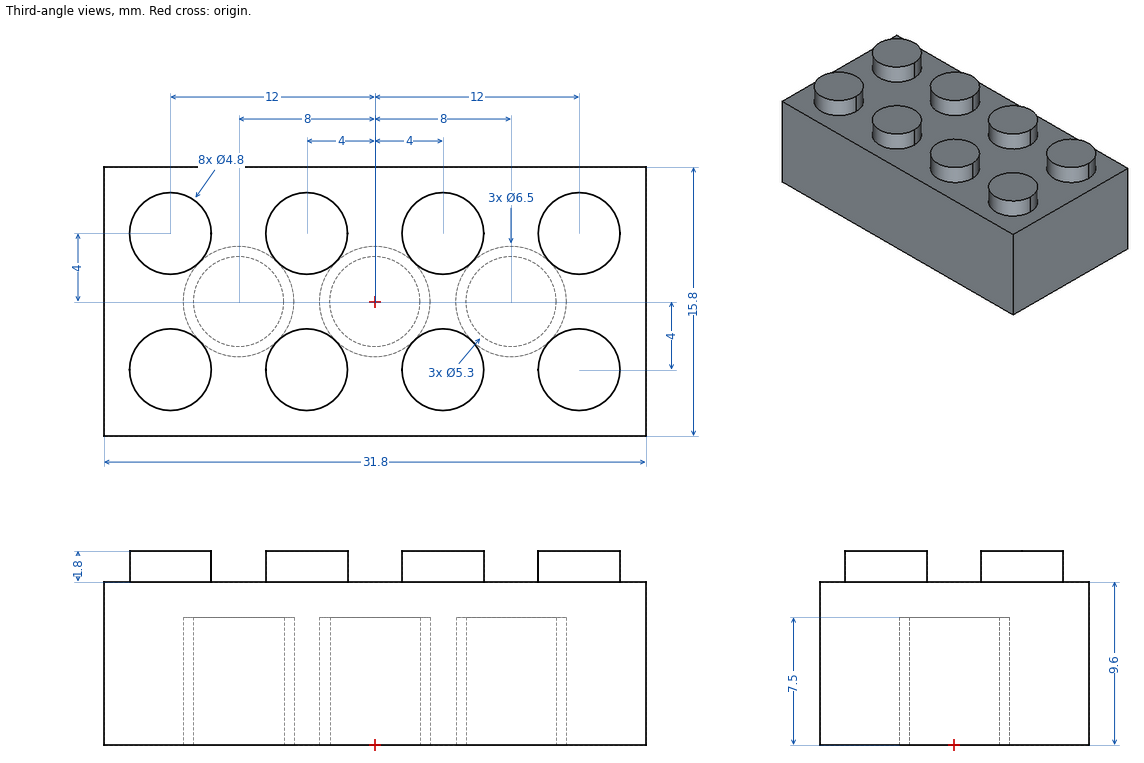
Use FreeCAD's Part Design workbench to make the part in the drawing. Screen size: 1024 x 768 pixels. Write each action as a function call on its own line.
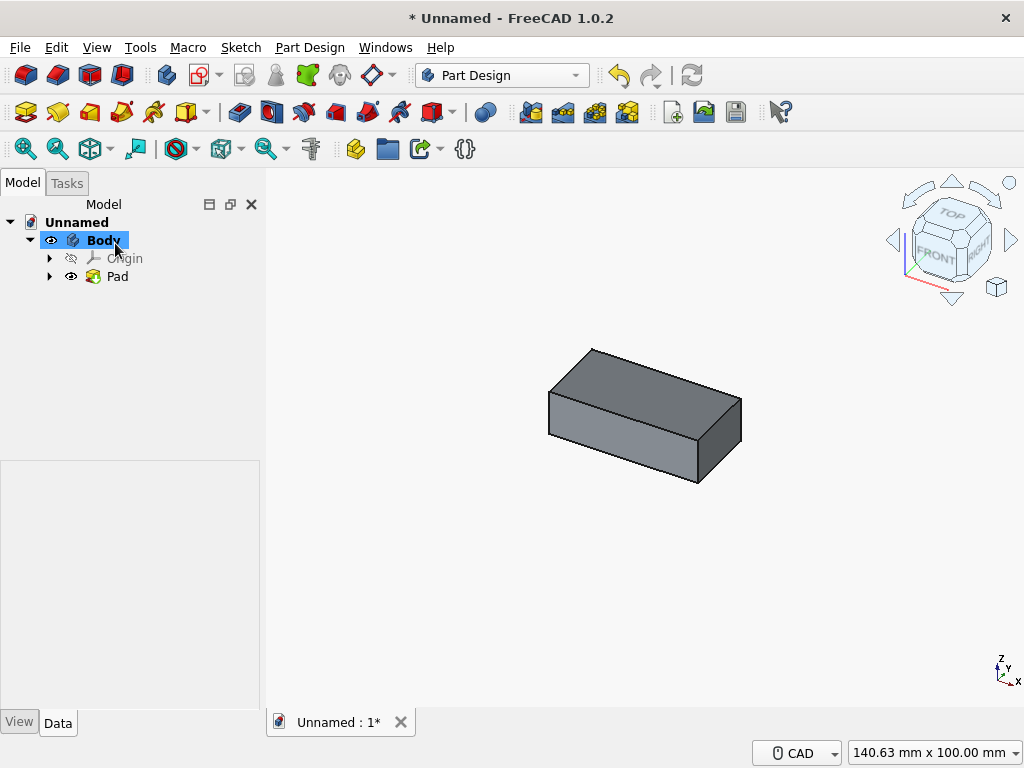
click(26, 150)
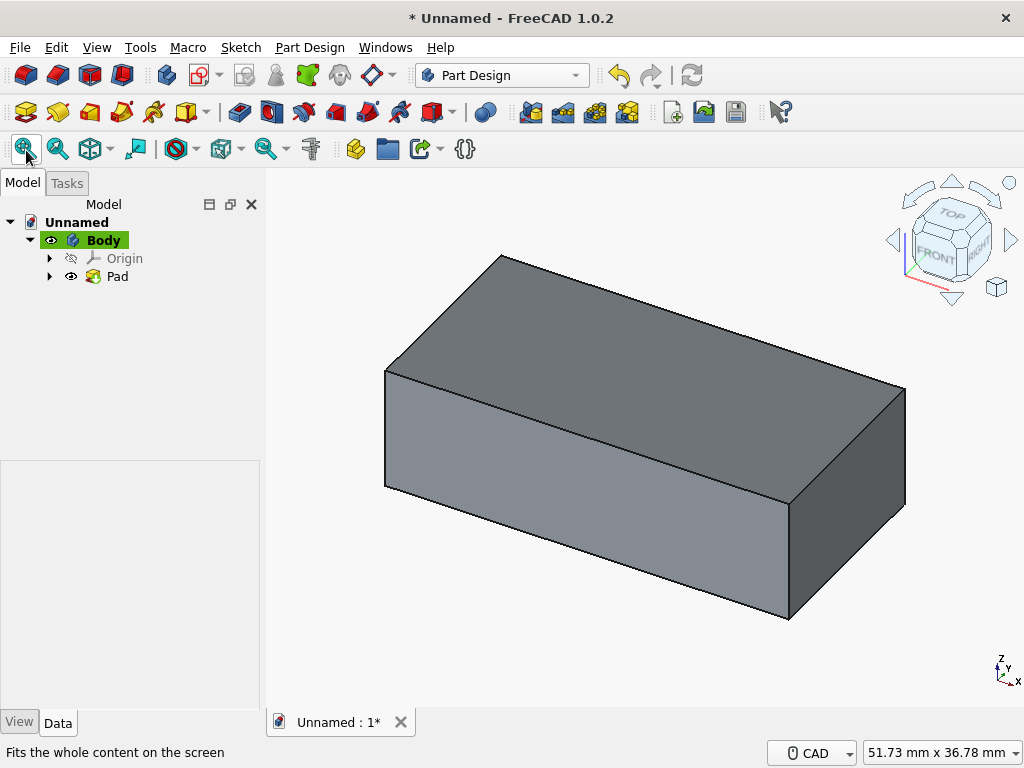
click(703, 398)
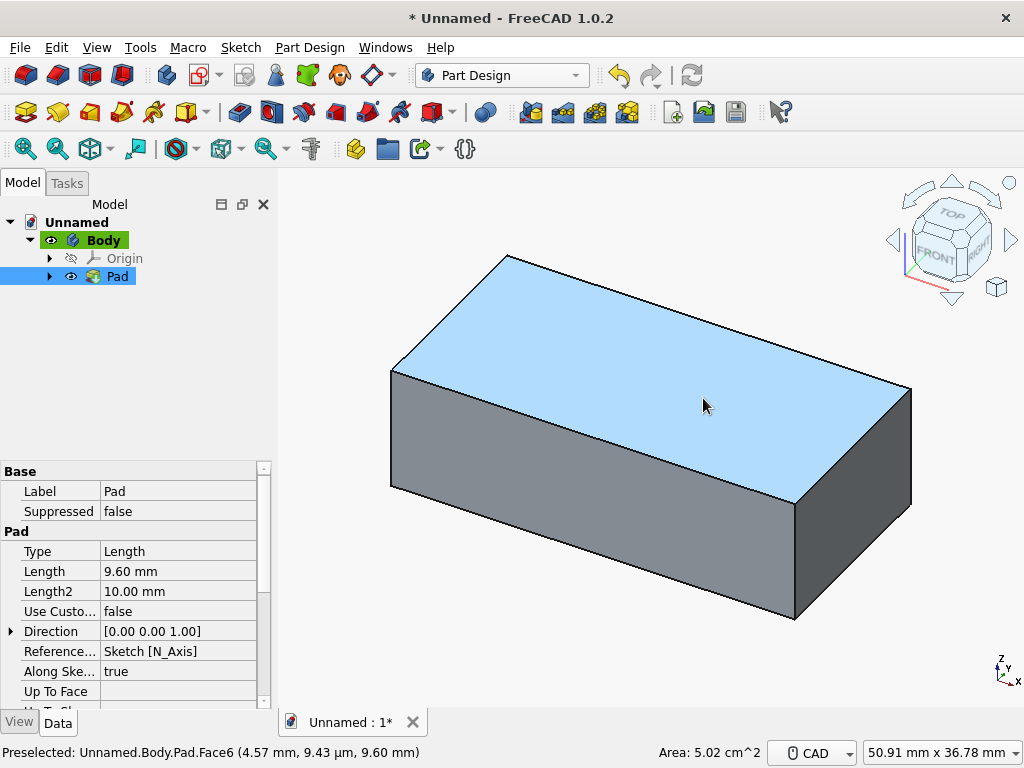
click(200, 76)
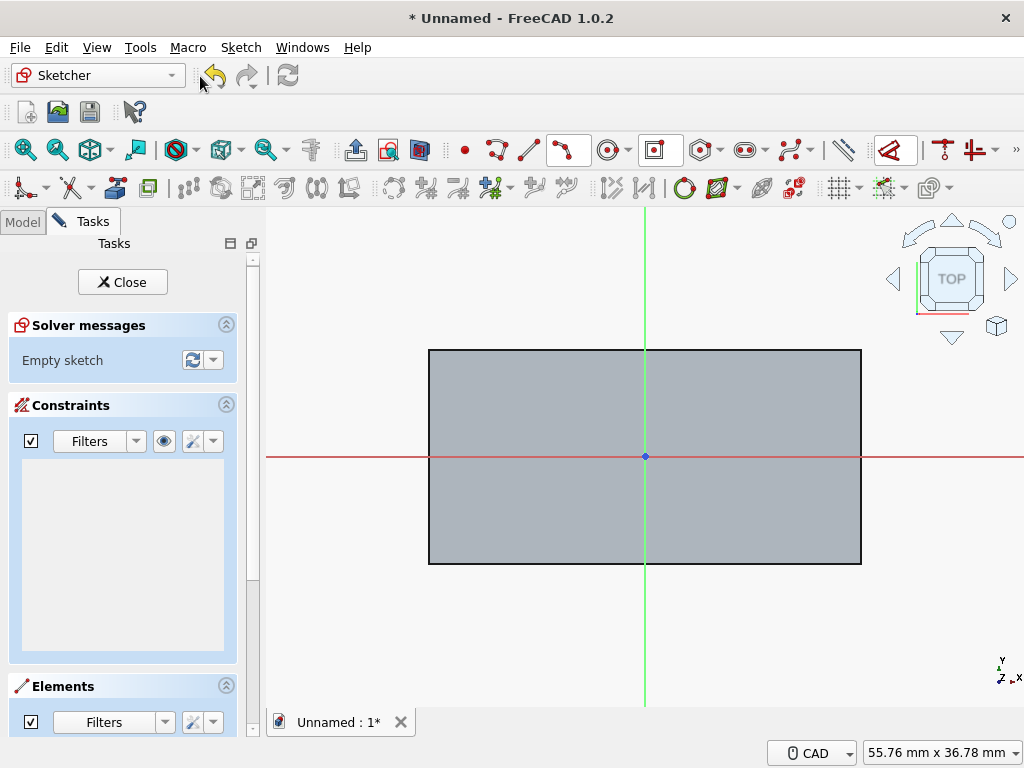
scroll(294, 457, down, 1)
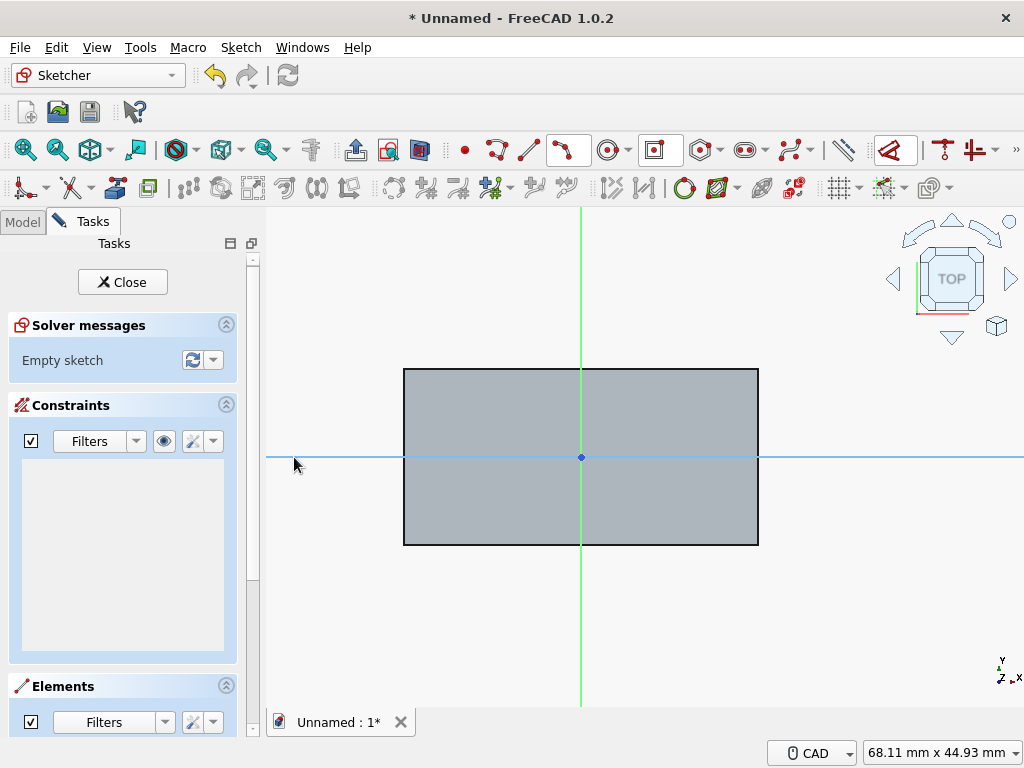
click(608, 150)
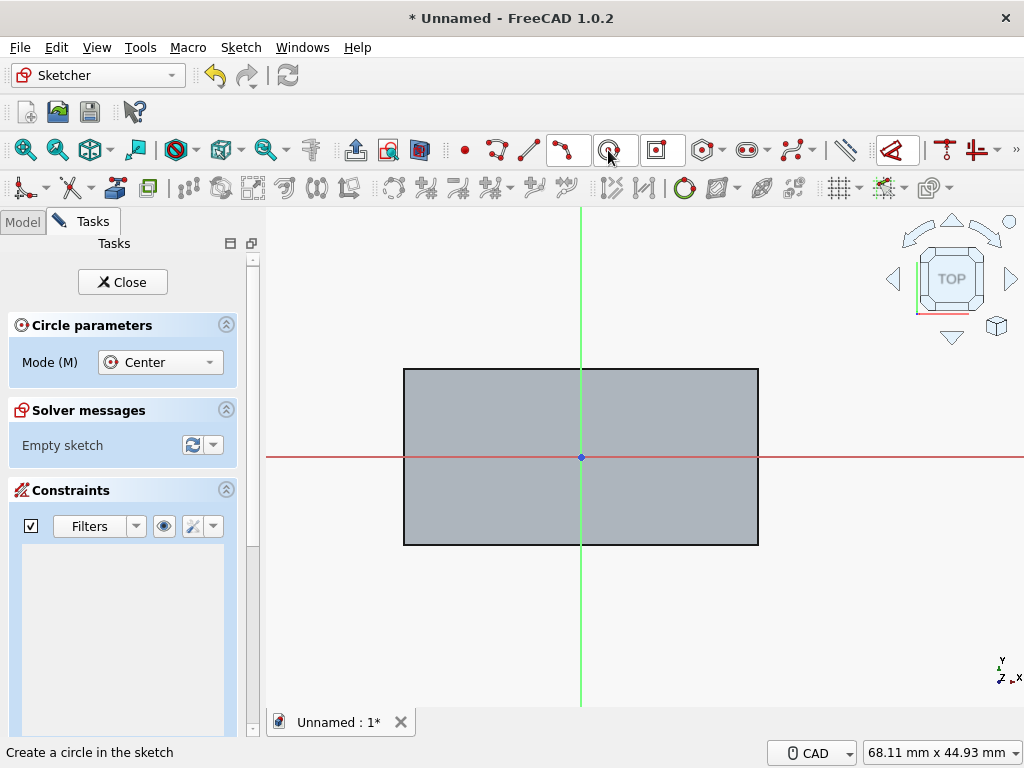
click(448, 413)
move(467, 394)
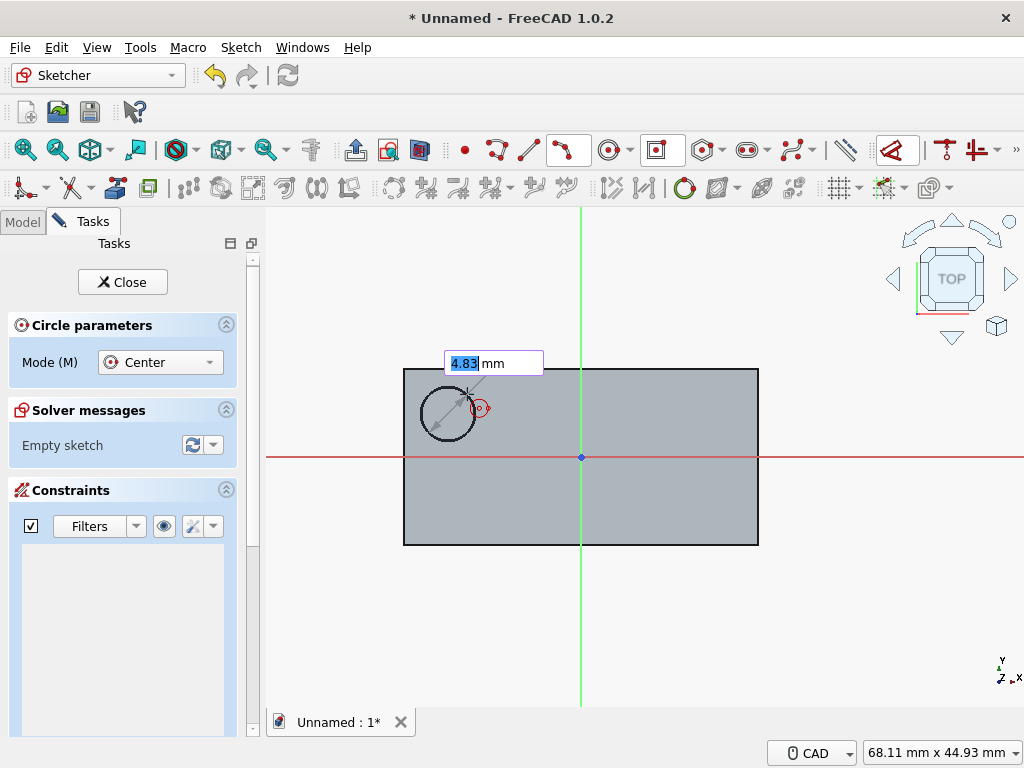
text(4.8)
key(Return)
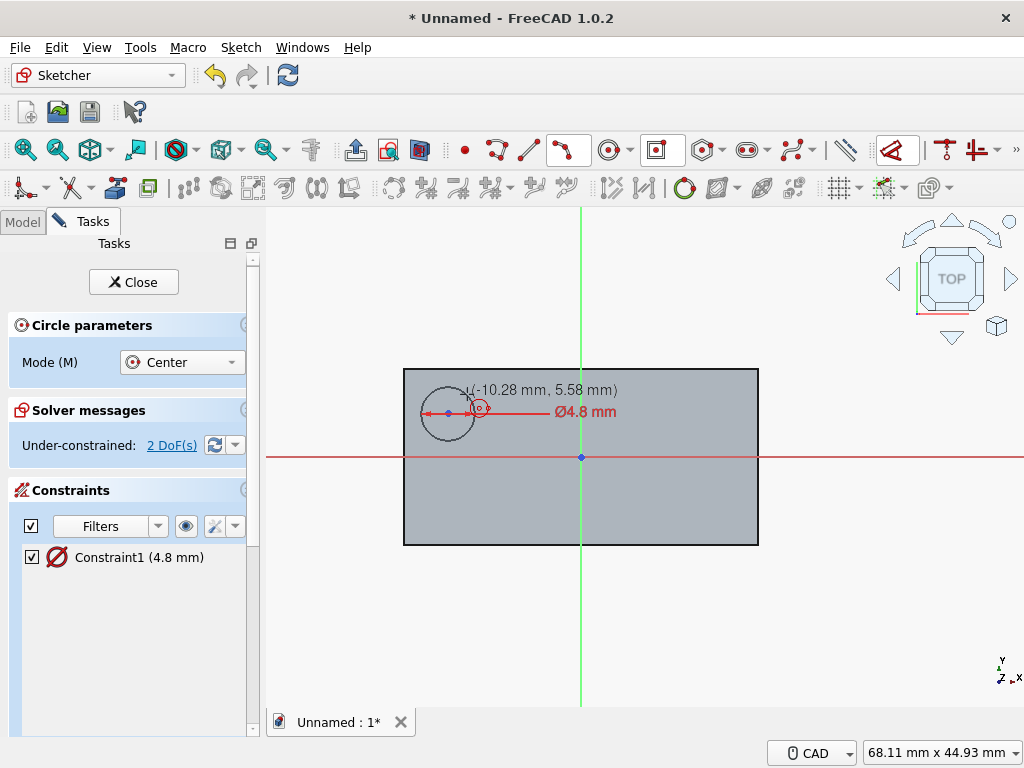
click(537, 413)
move(556, 394)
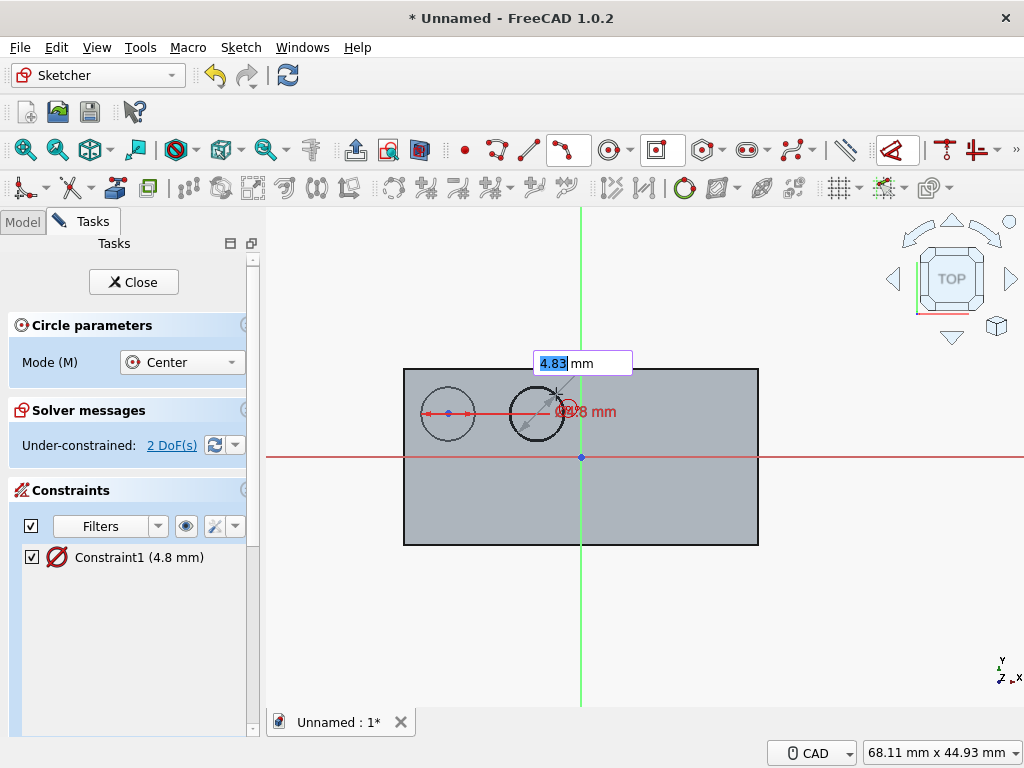
text(4.8)
key(Return)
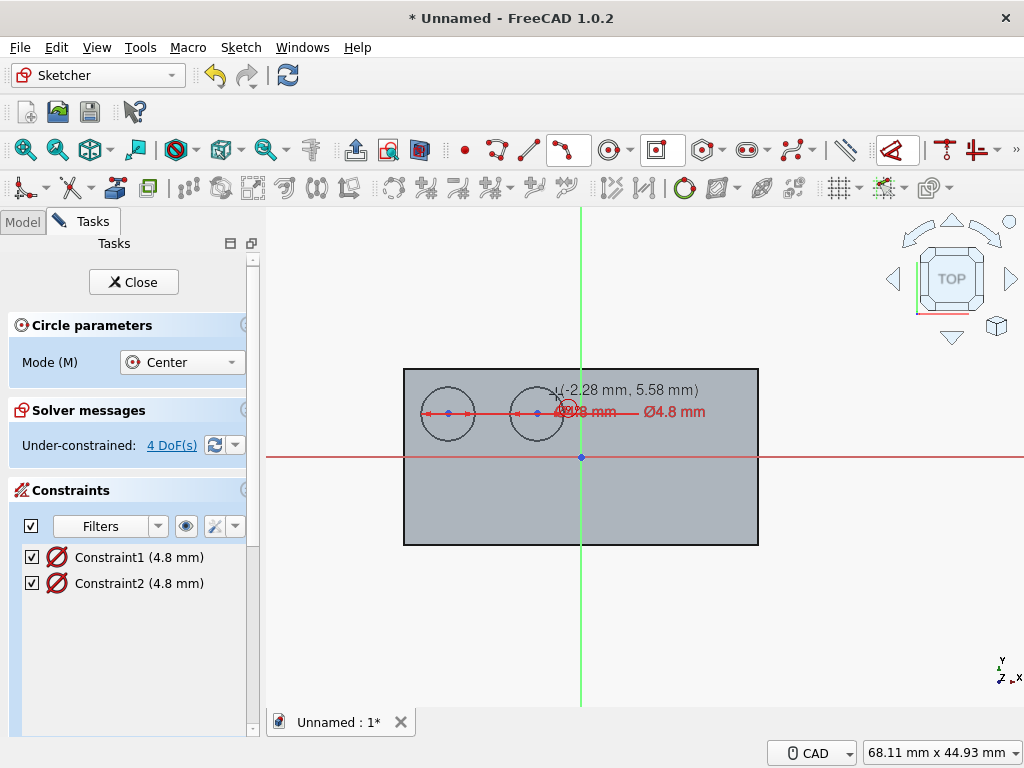
click(626, 413)
move(645, 394)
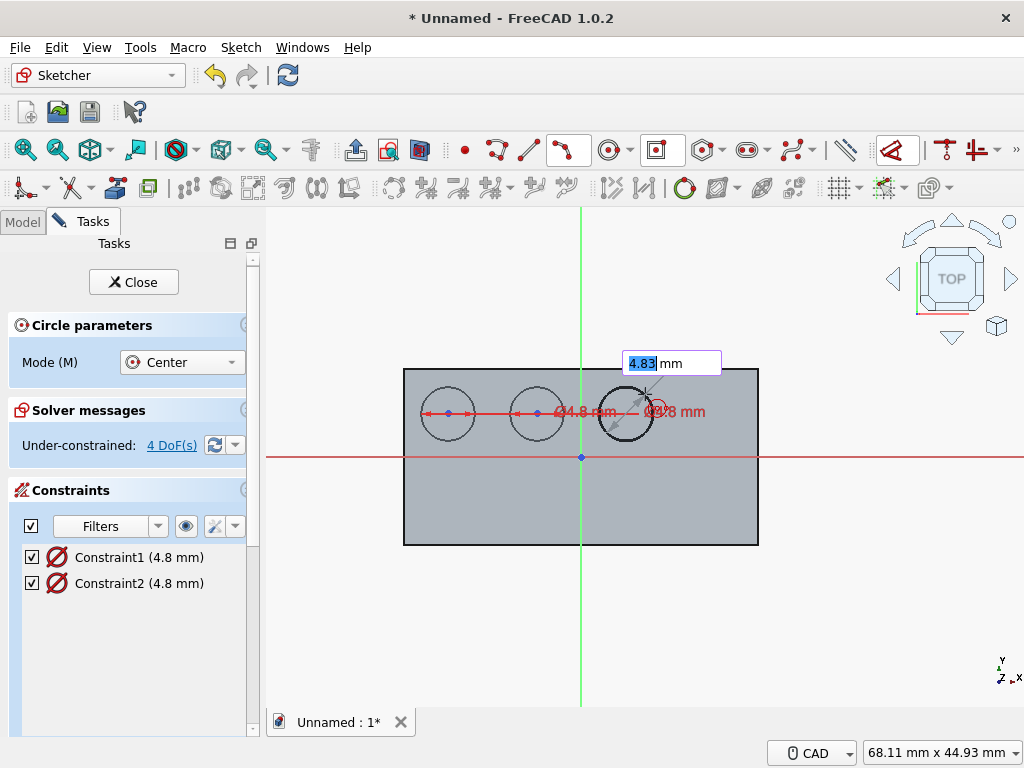
text(4.8)
key(Return)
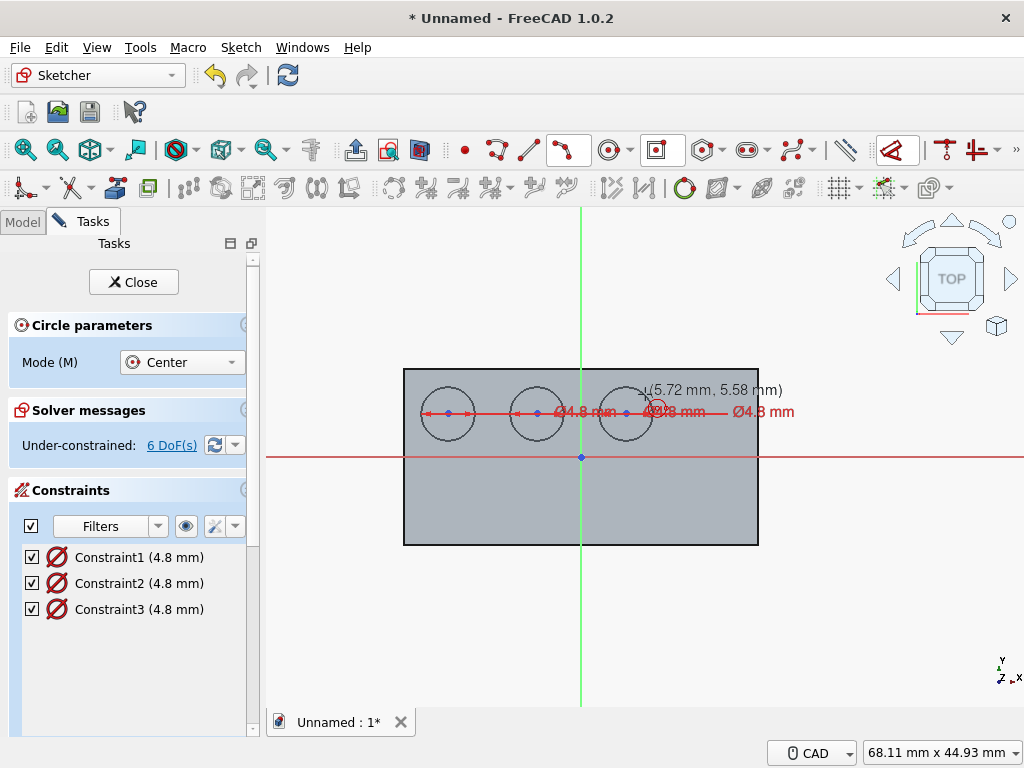
click(715, 413)
move(734, 394)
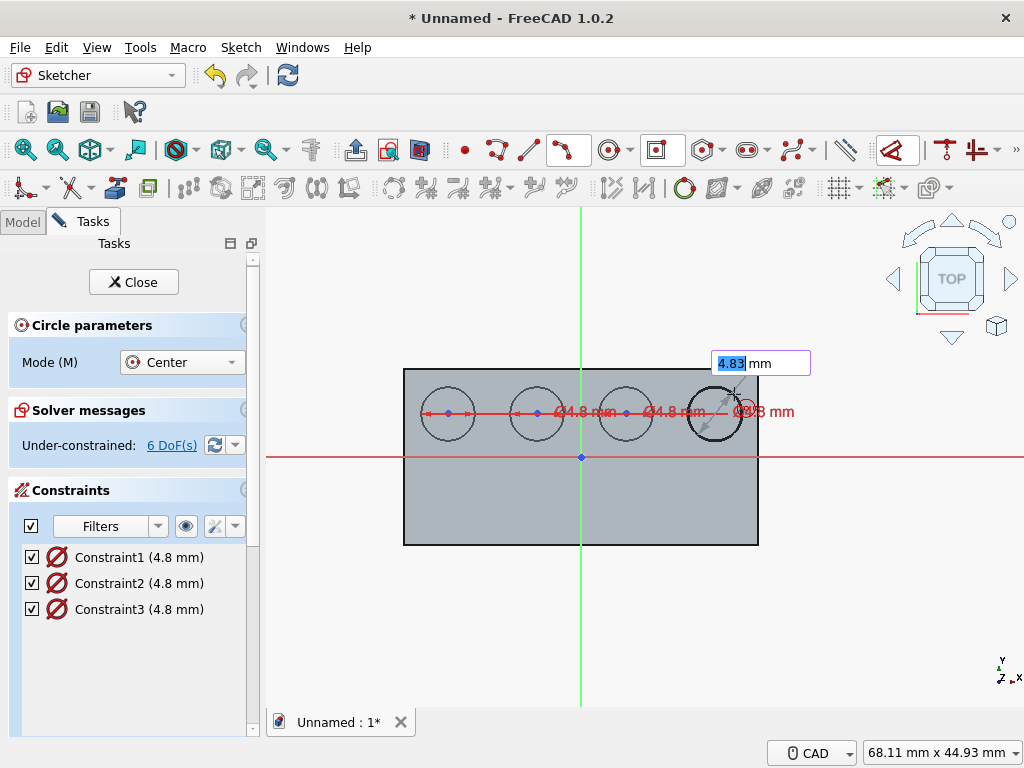
text(4.8)
key(Return)